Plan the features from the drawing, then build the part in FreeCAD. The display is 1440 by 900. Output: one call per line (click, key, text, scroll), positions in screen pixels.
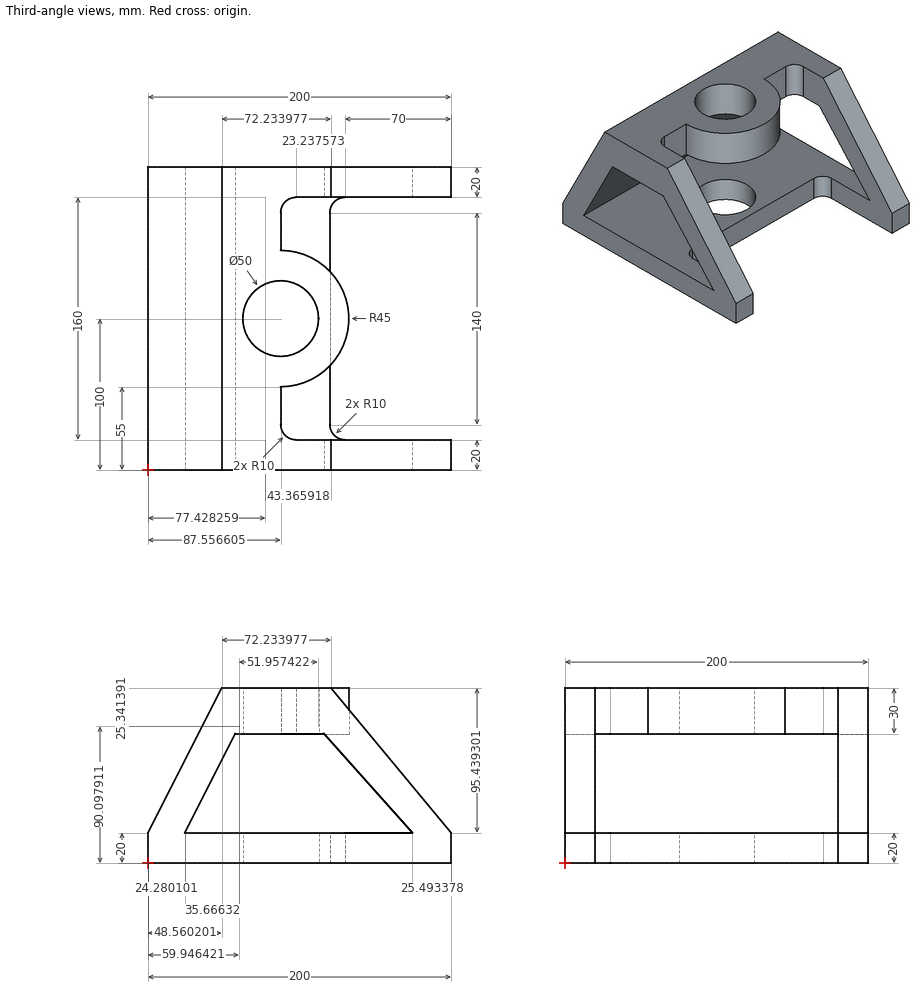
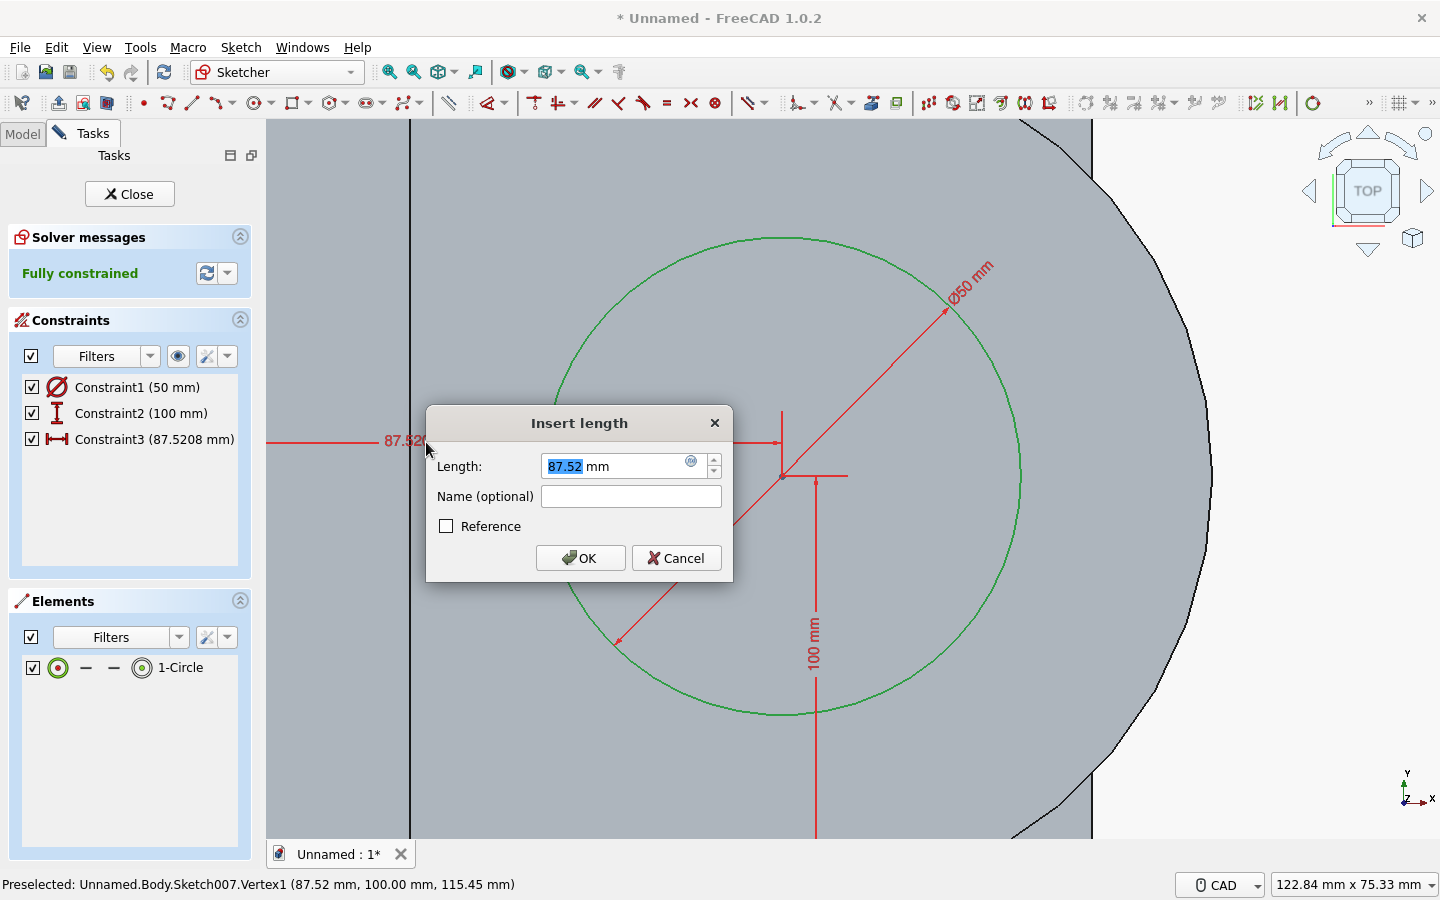
text(87.556605)
key(Return)
key(Escape)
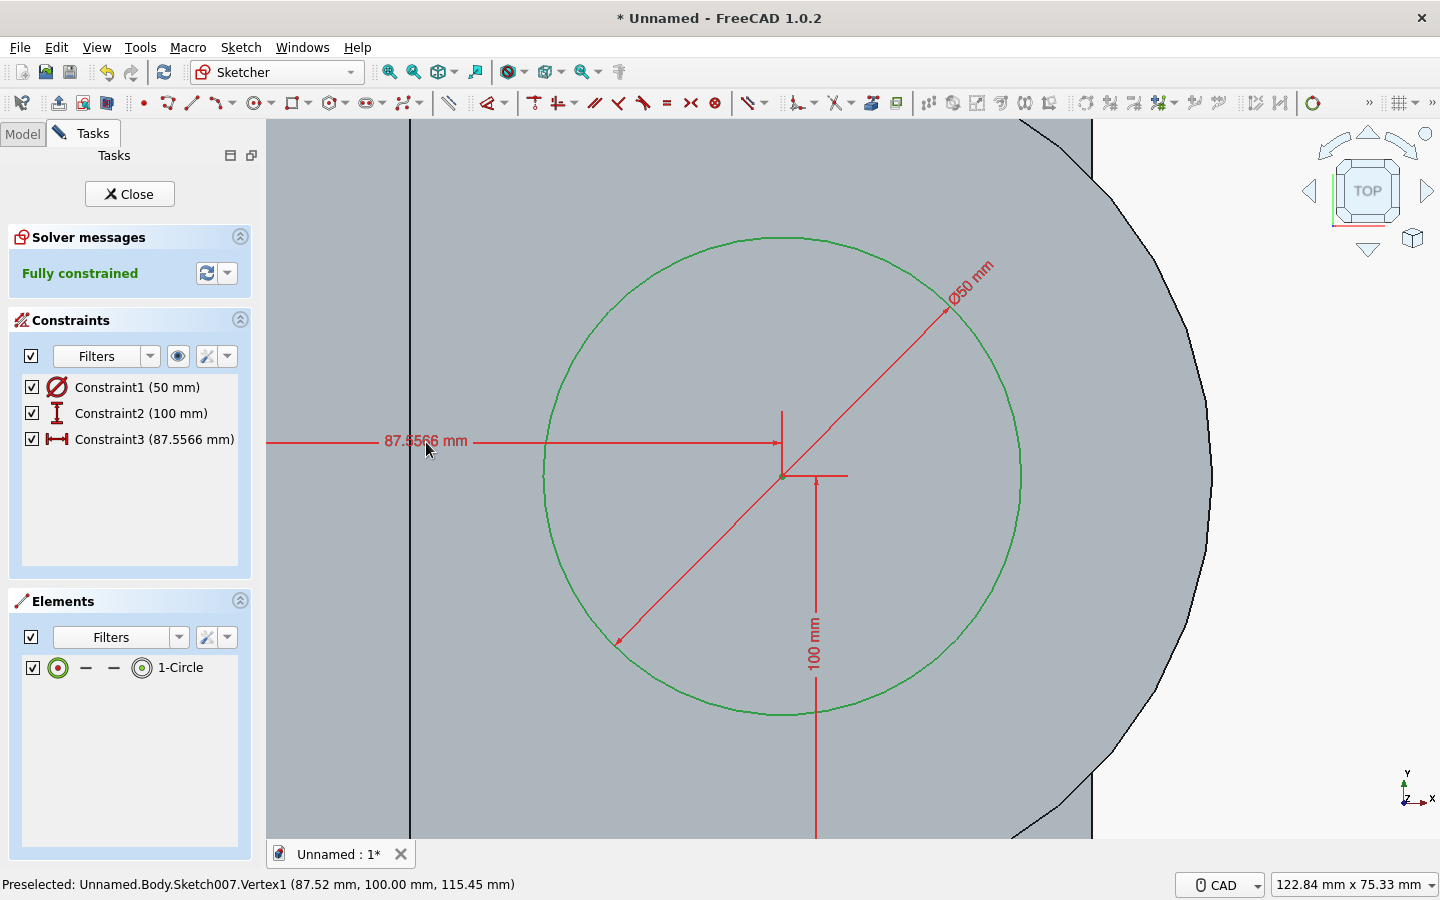
click(130, 194)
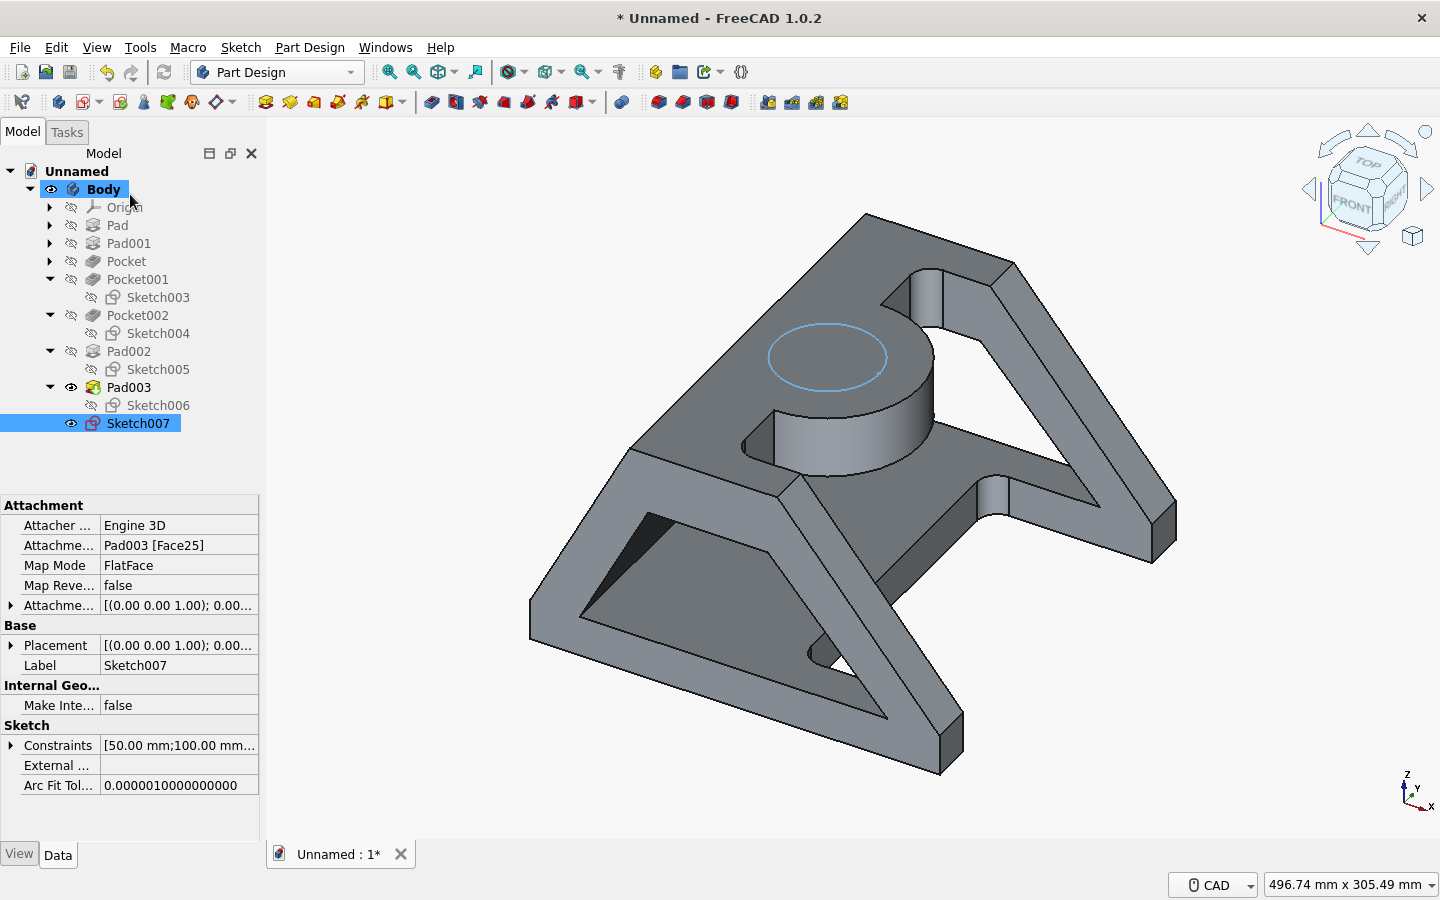
click(432, 102)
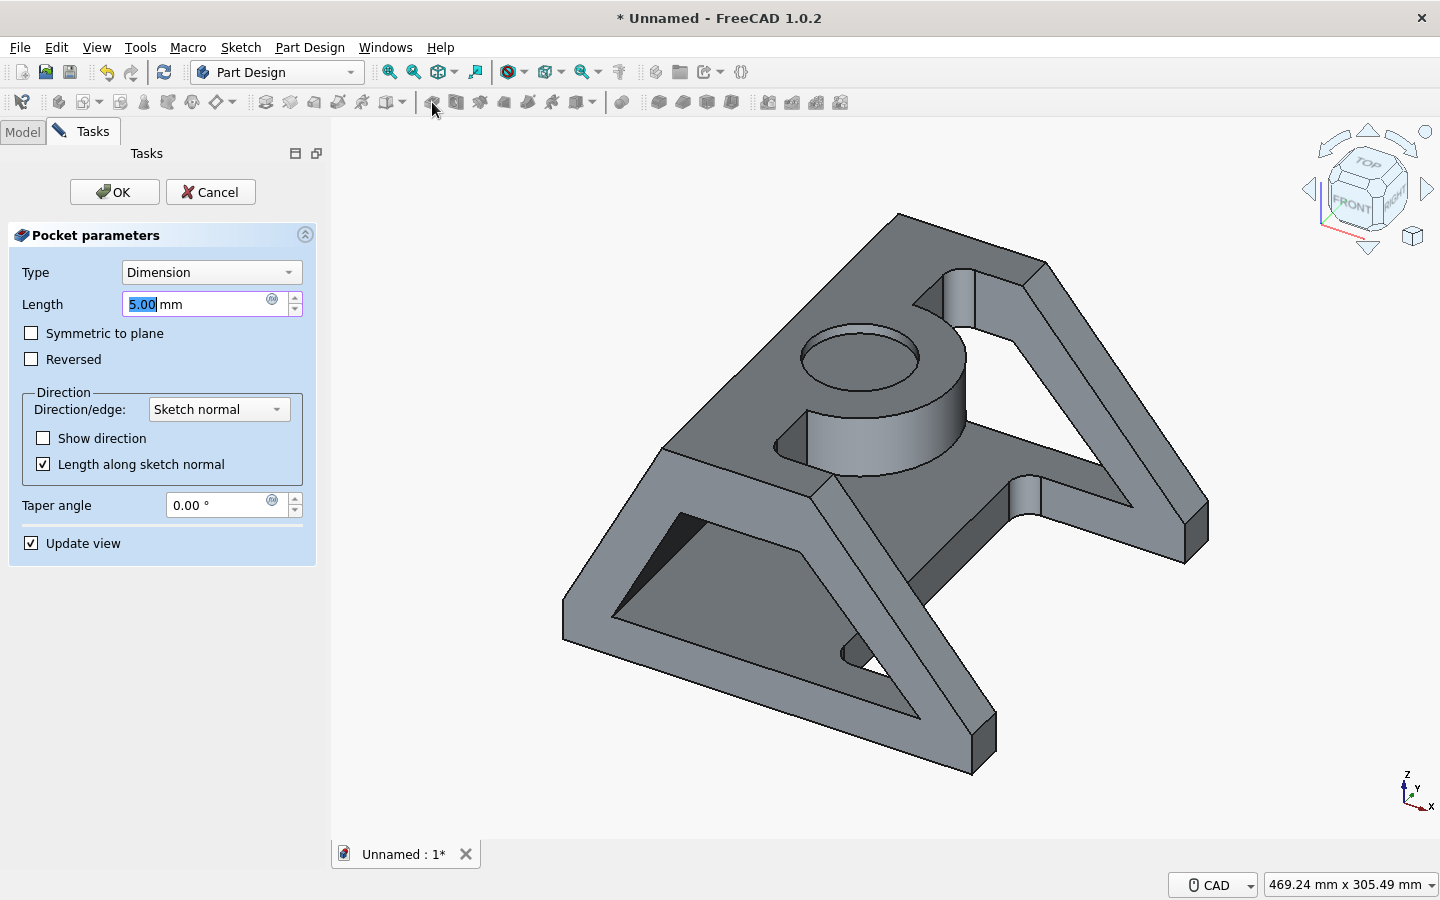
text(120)
key(Tab)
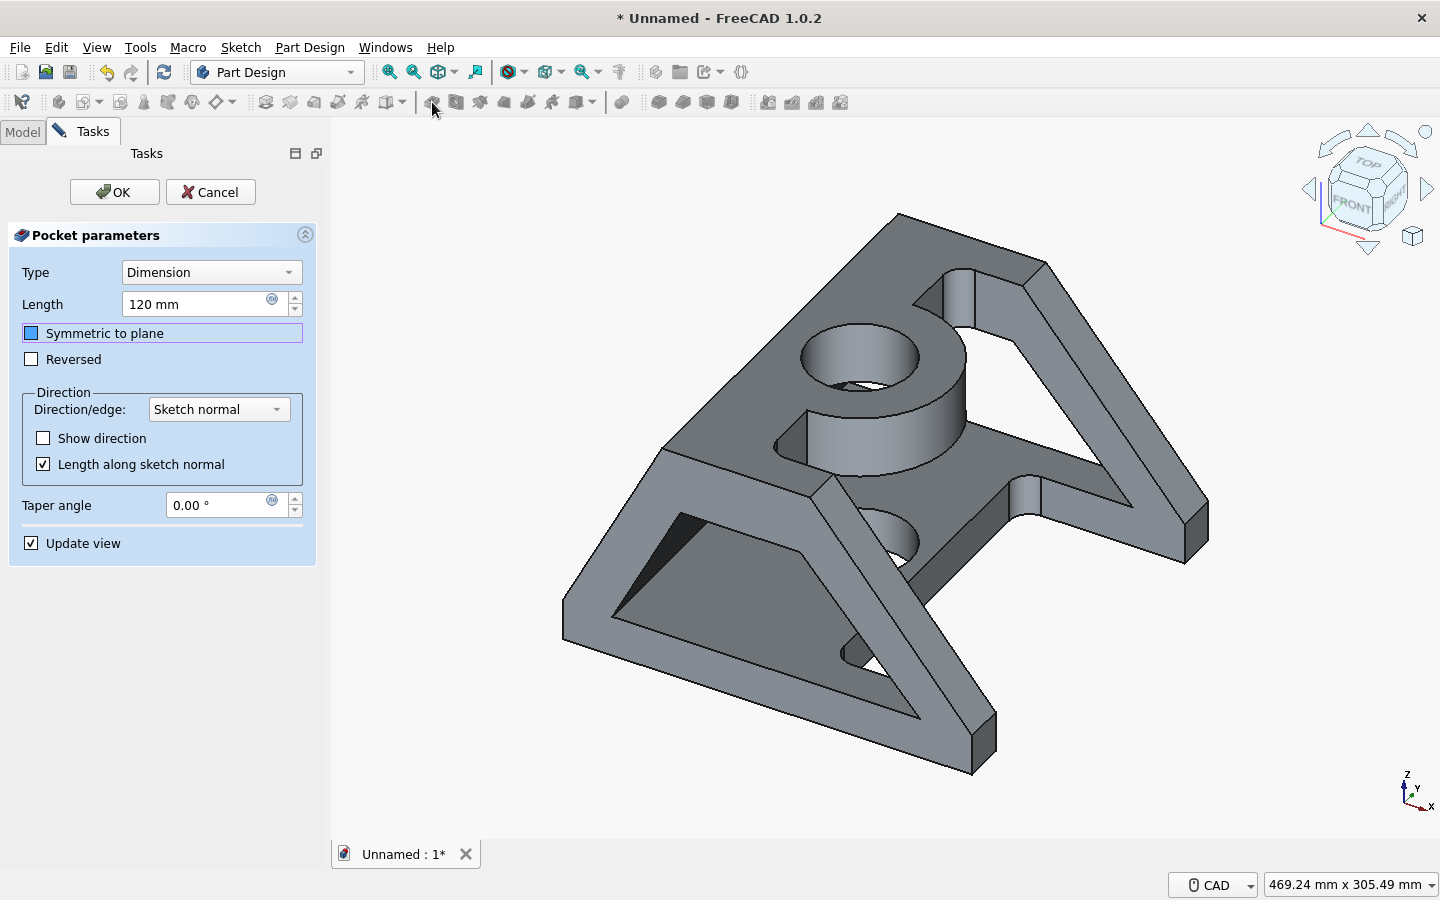
click(115, 192)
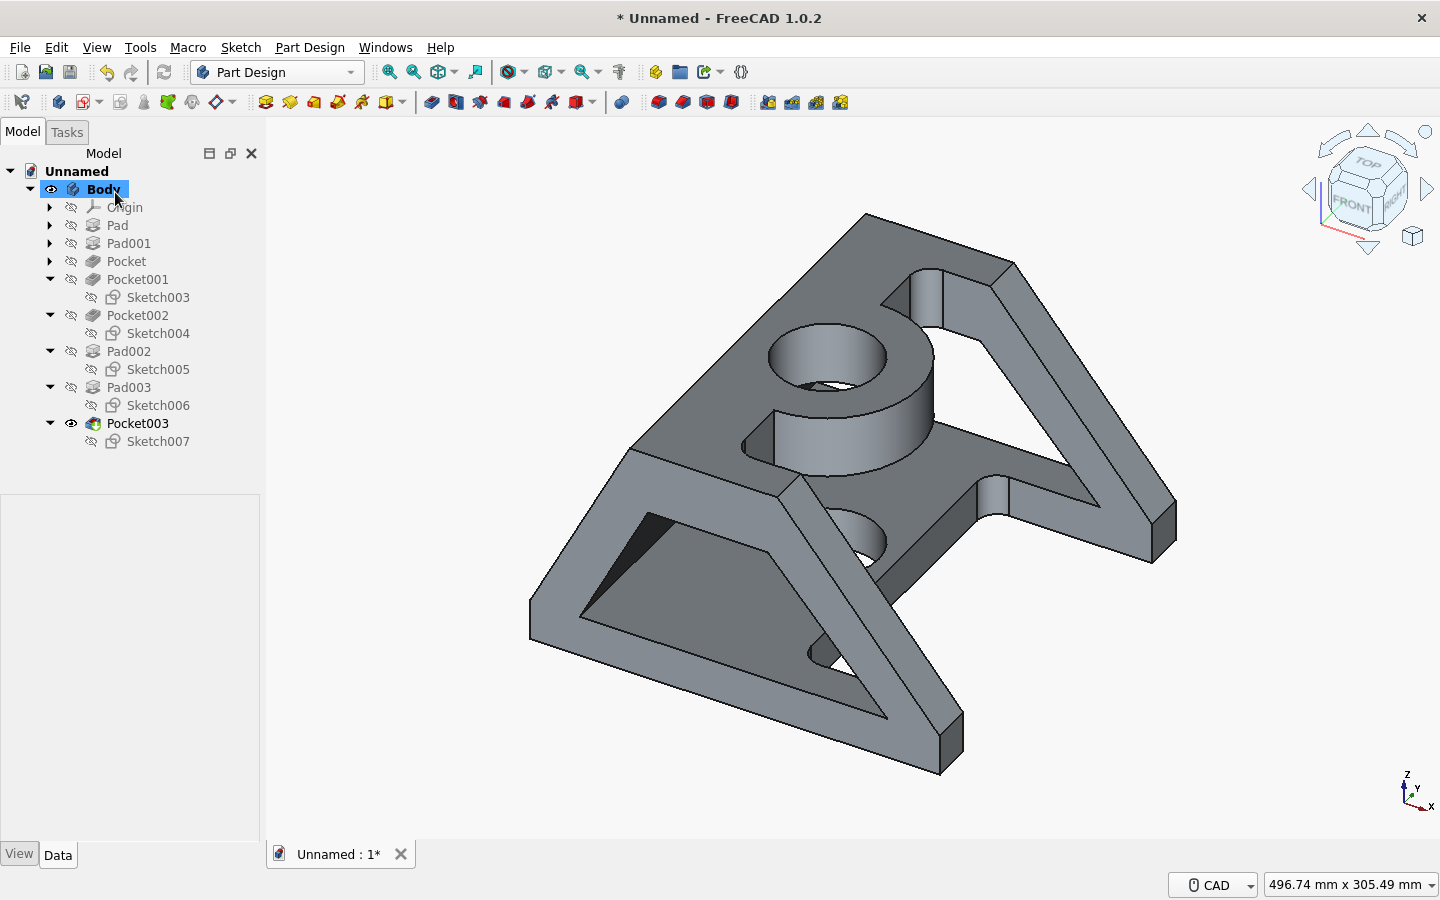
key(0)